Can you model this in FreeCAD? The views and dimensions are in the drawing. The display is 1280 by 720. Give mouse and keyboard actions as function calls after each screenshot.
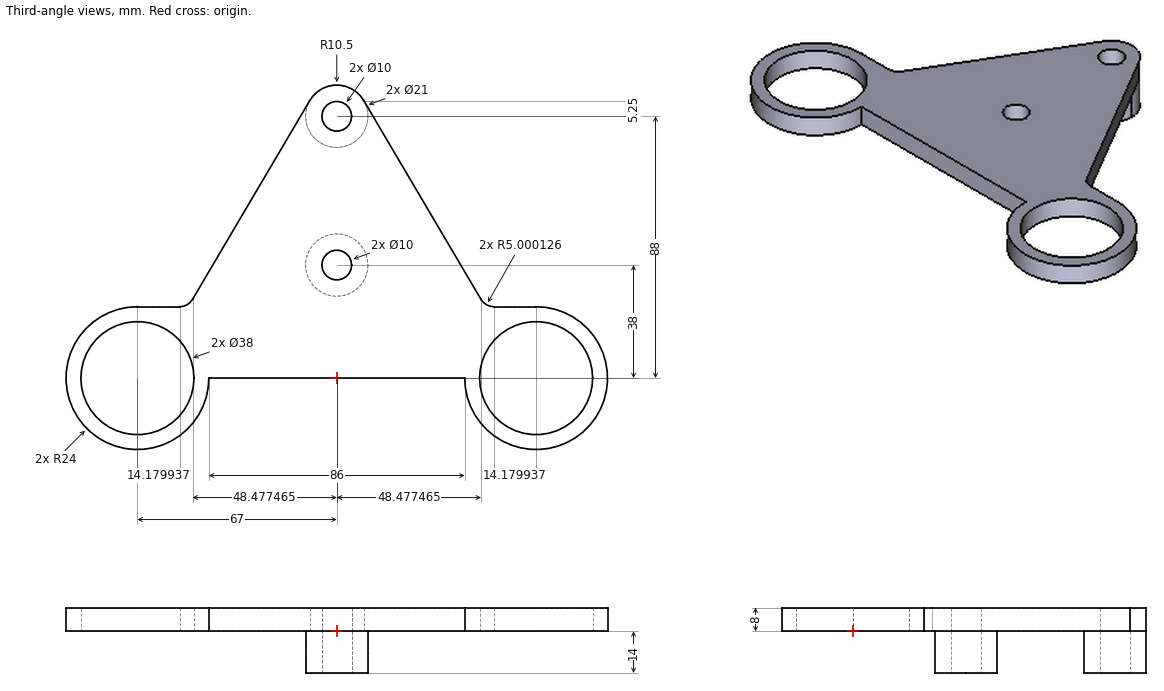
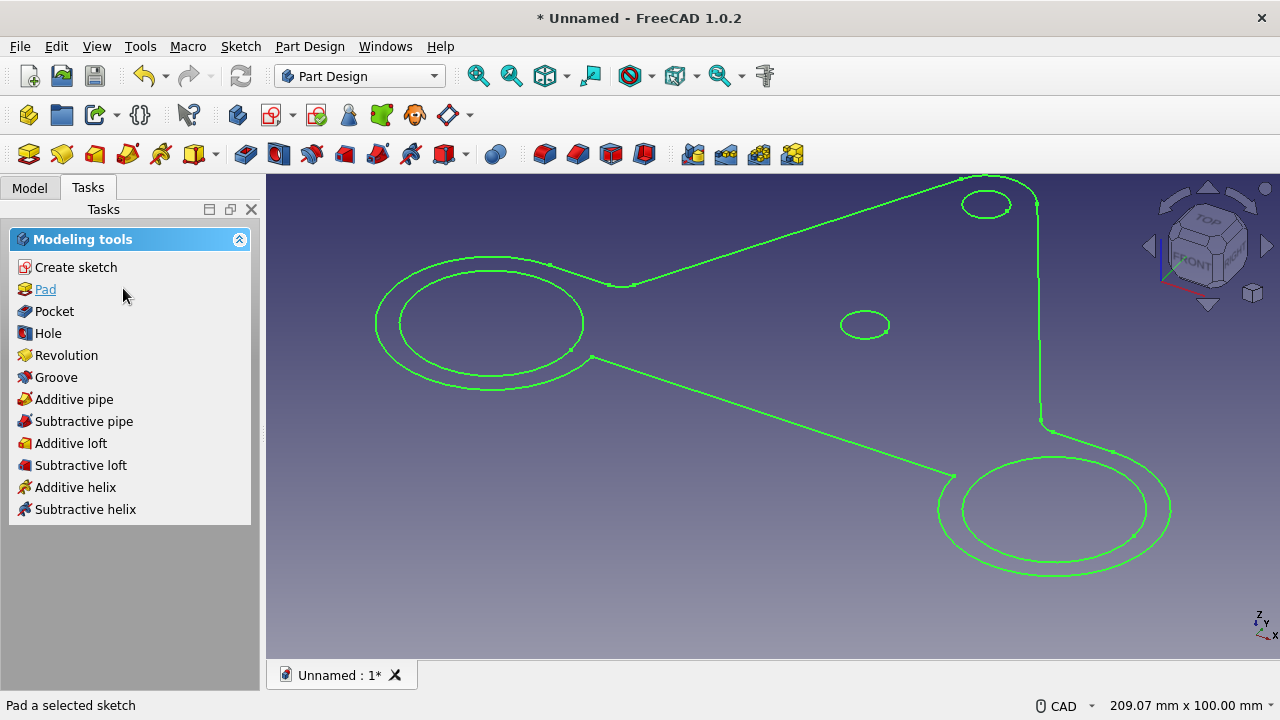
click(29, 154)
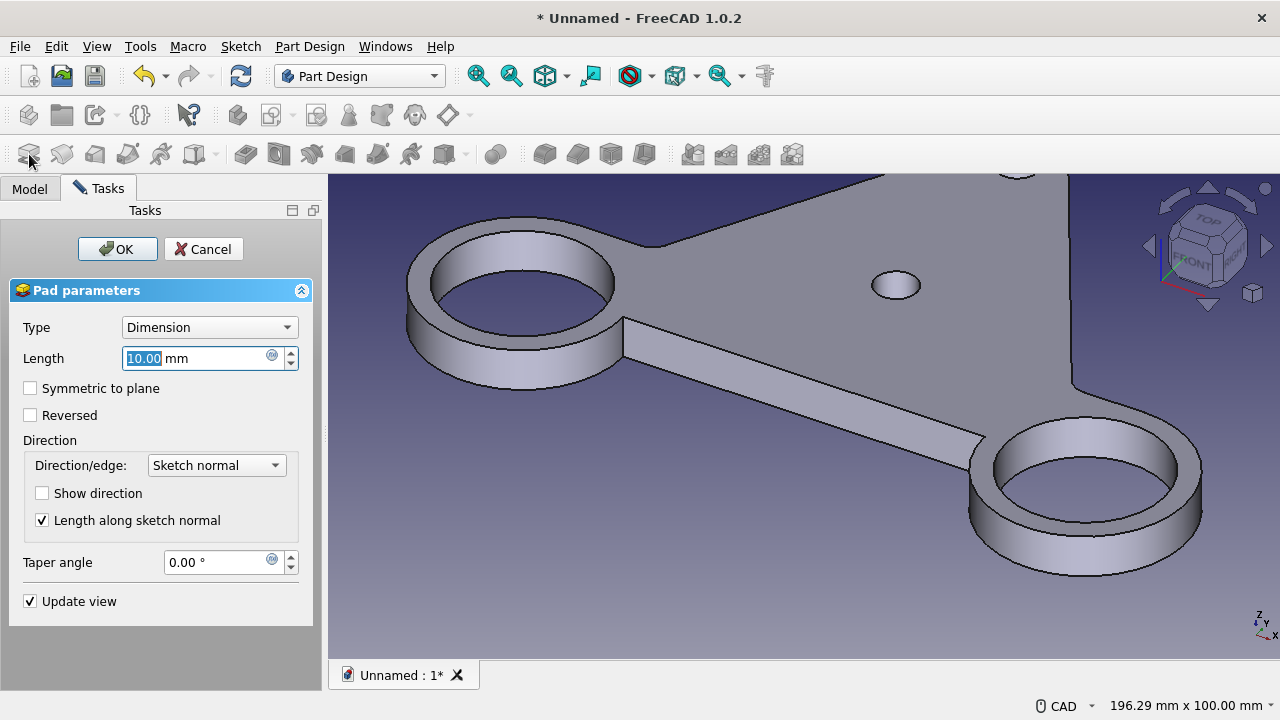
text(8)
key(Tab)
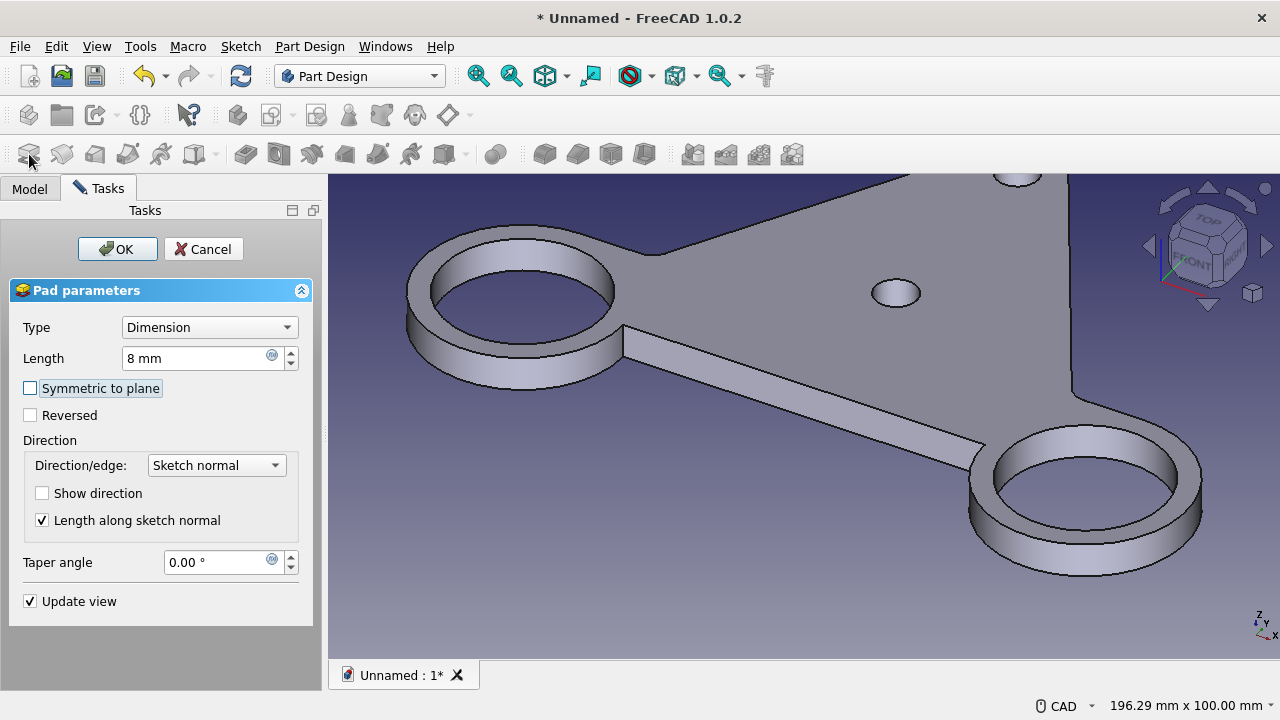
click(118, 249)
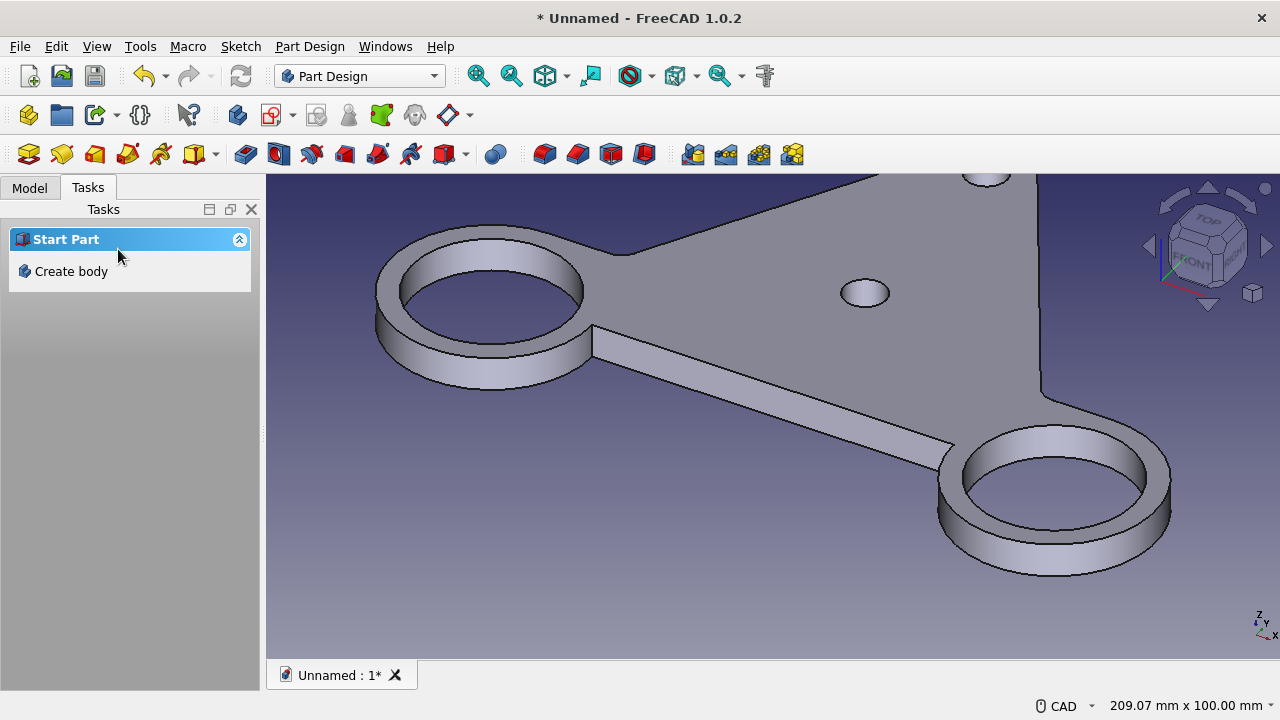
click(479, 76)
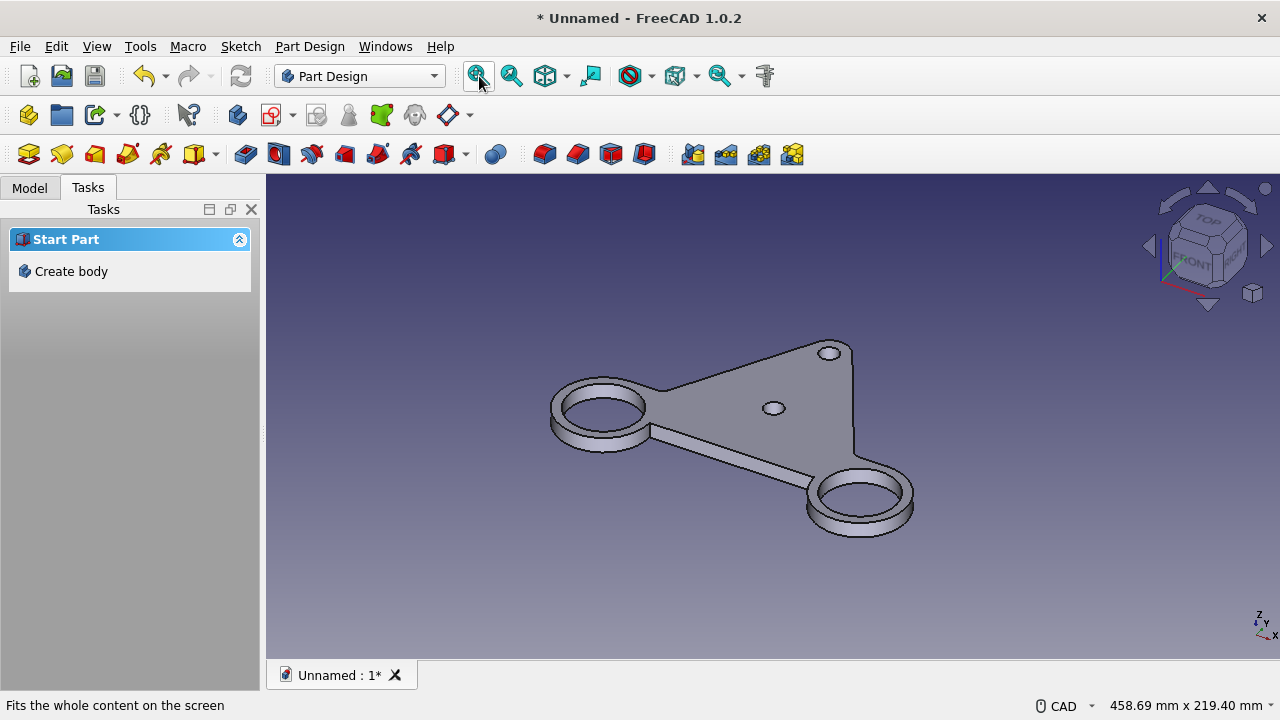
click(30, 188)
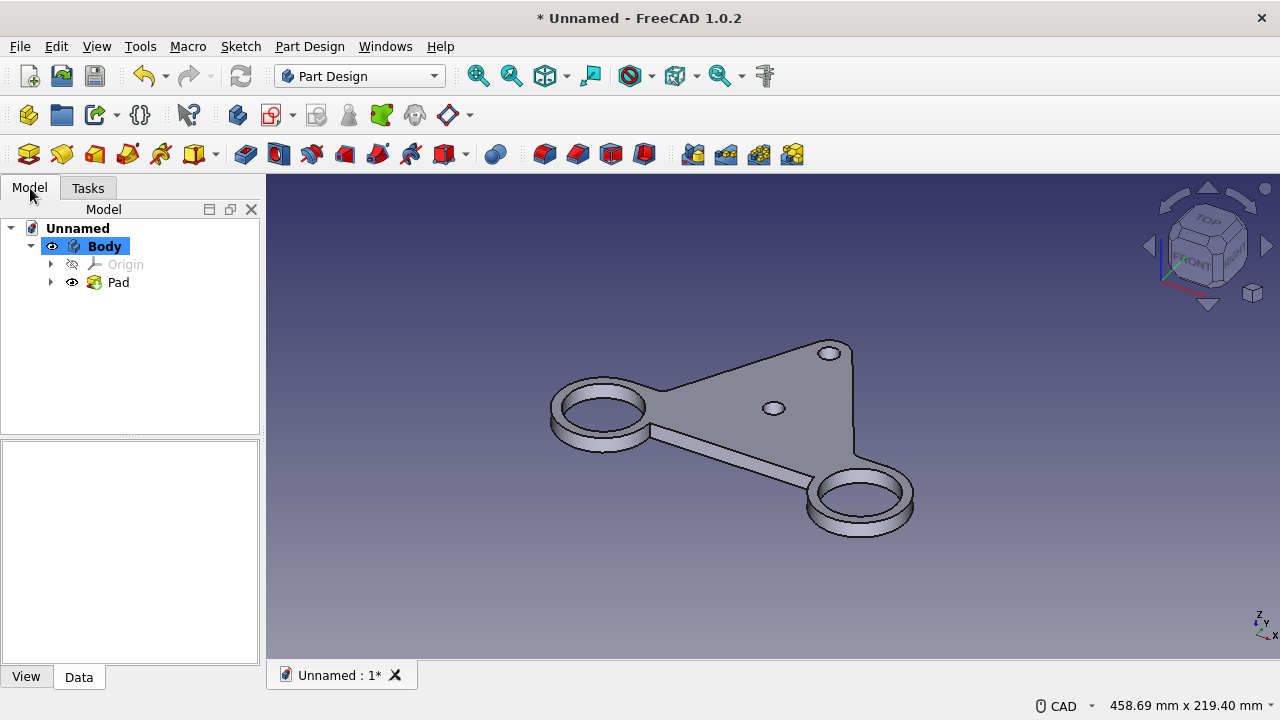
click(51, 264)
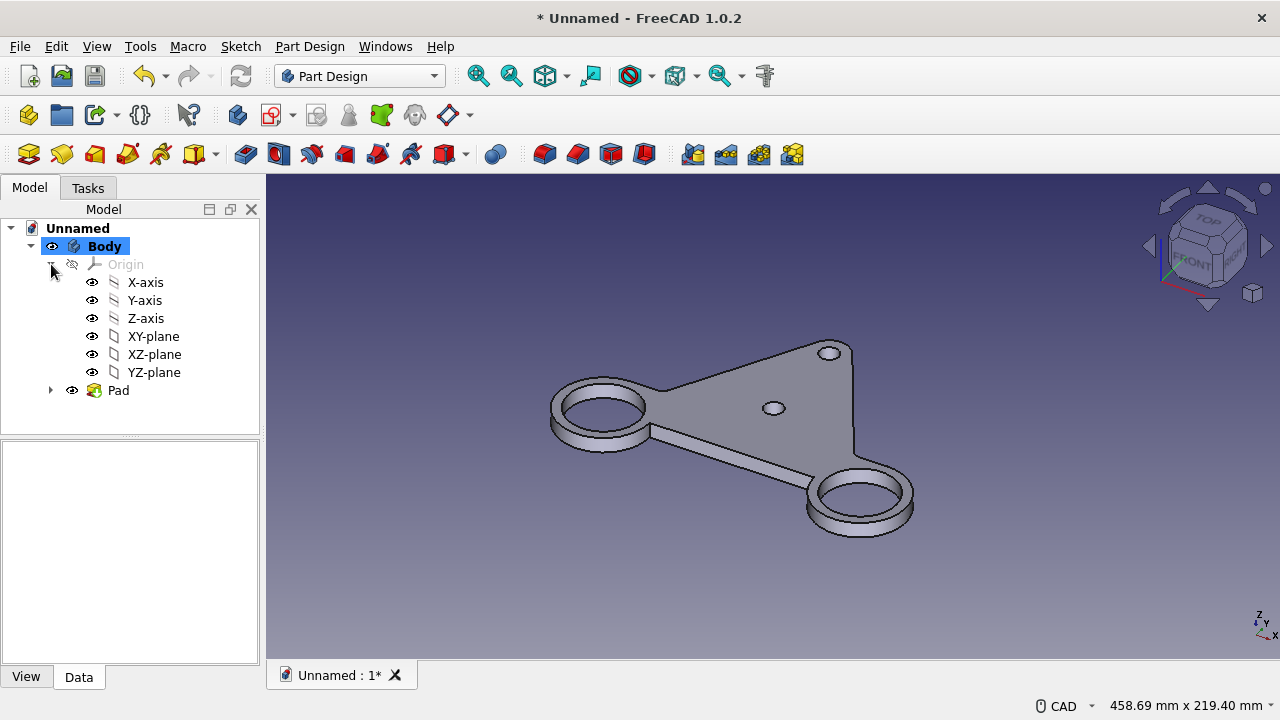
click(137, 336)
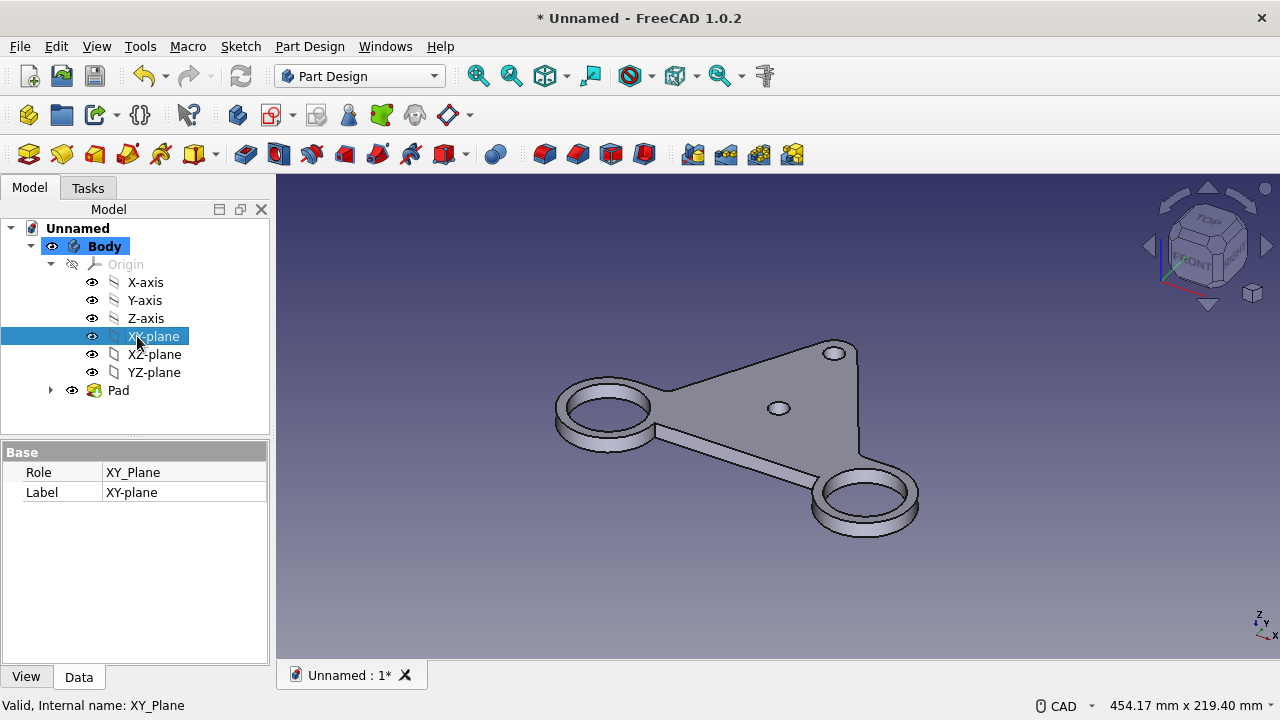
click(448, 116)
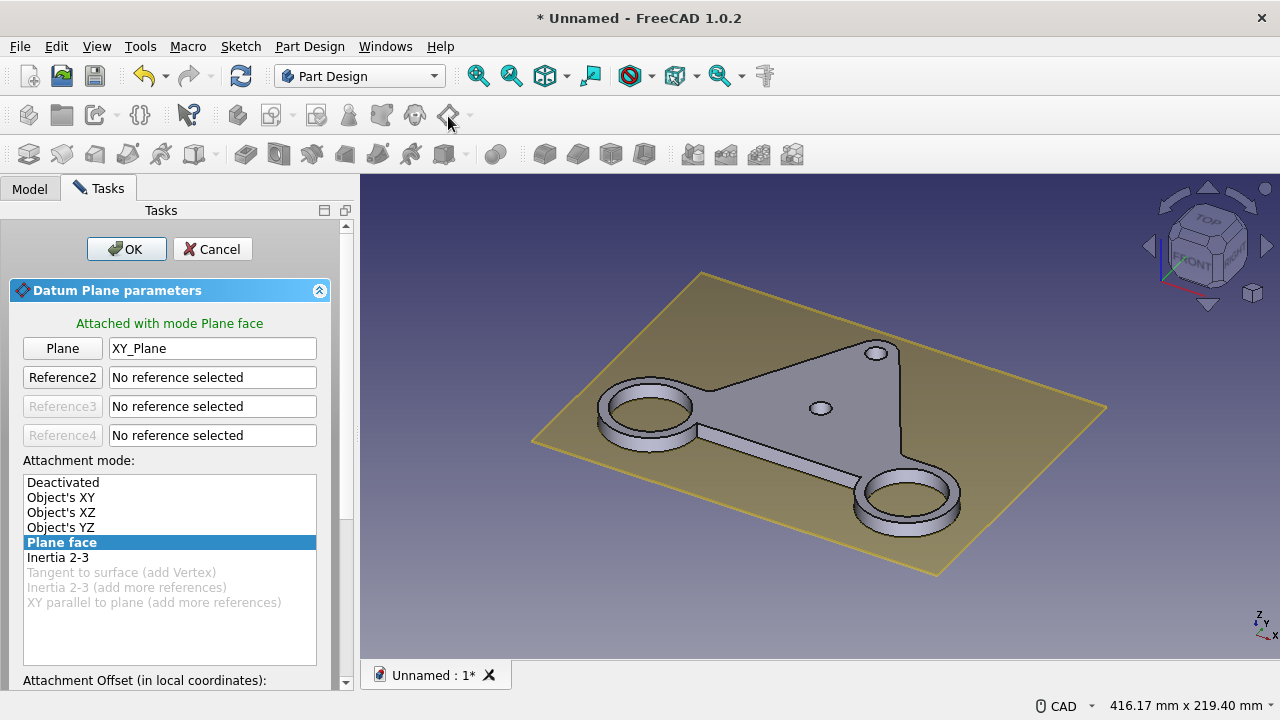
scroll(346, 455, down, 3)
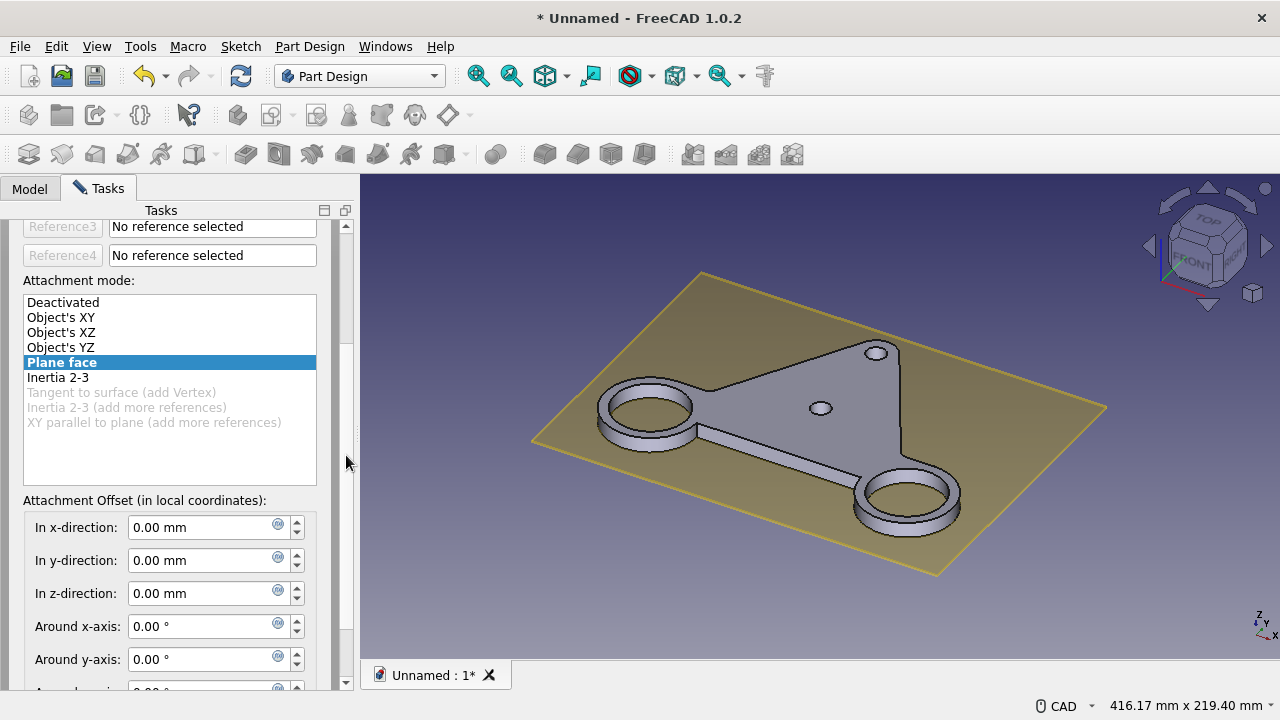
triple_click(210, 594)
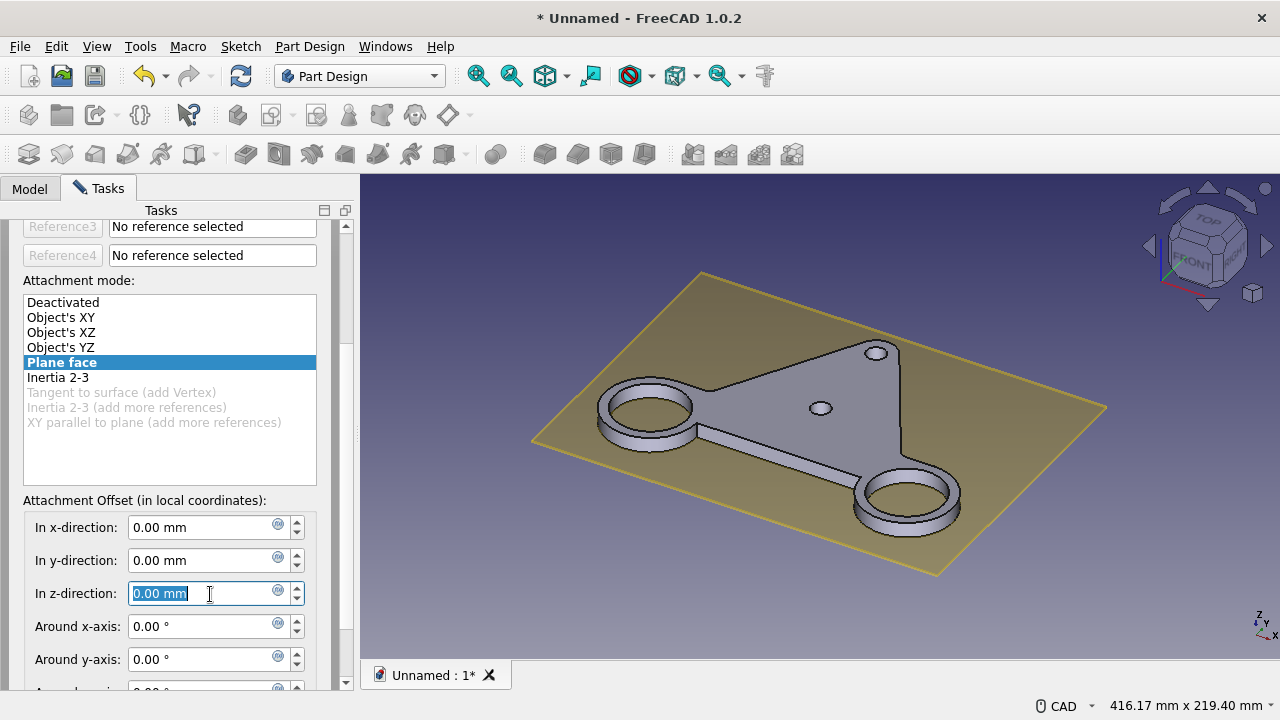
text(-14)
key(Tab)